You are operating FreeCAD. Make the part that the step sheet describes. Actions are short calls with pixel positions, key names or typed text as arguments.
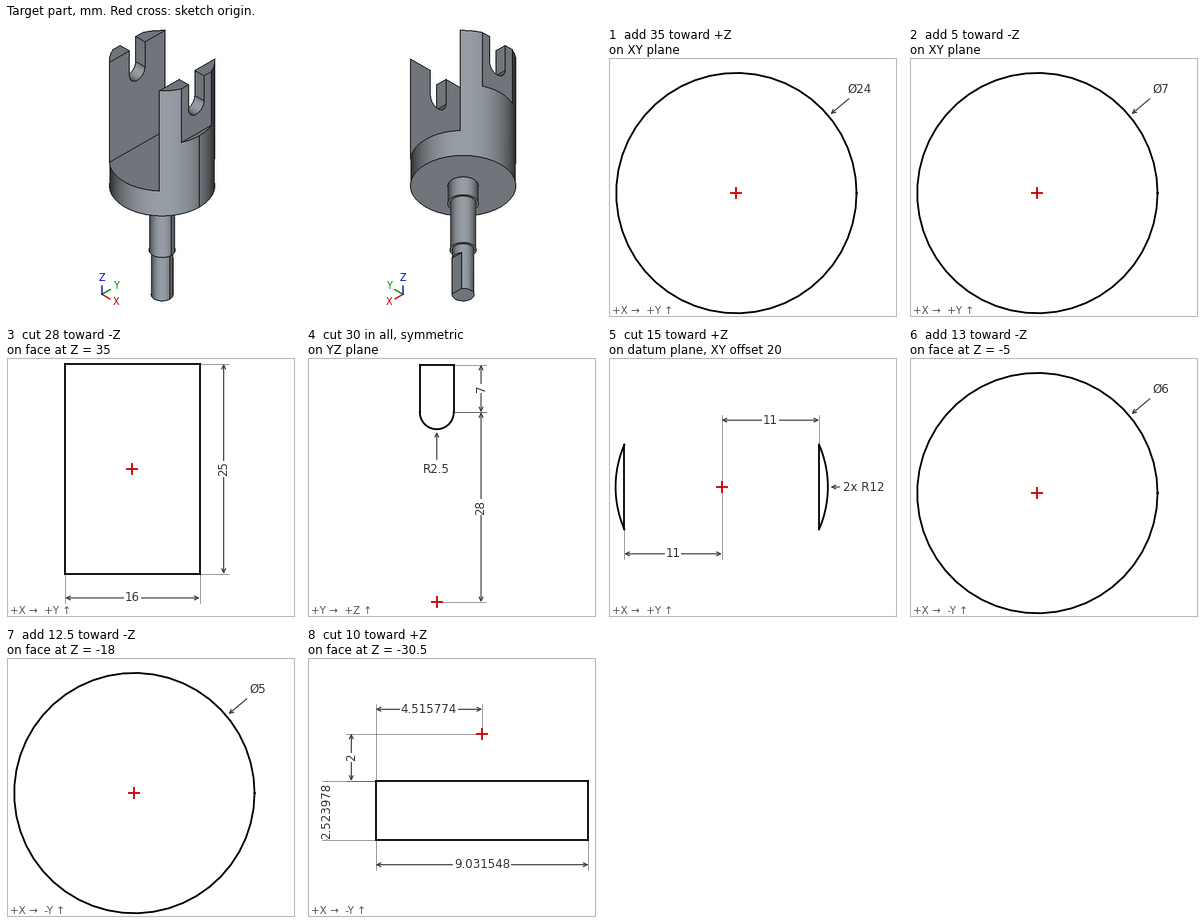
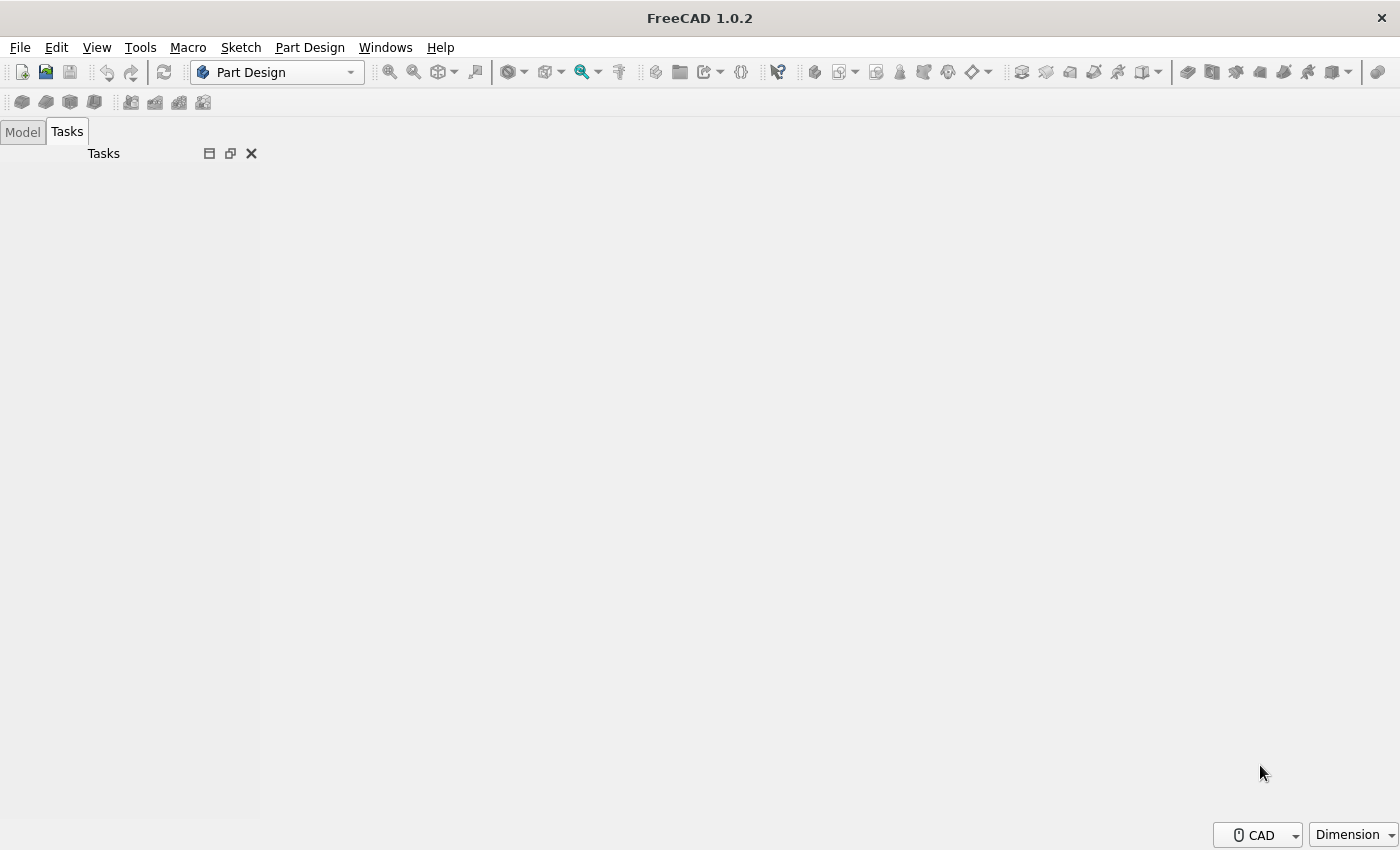
click(22, 72)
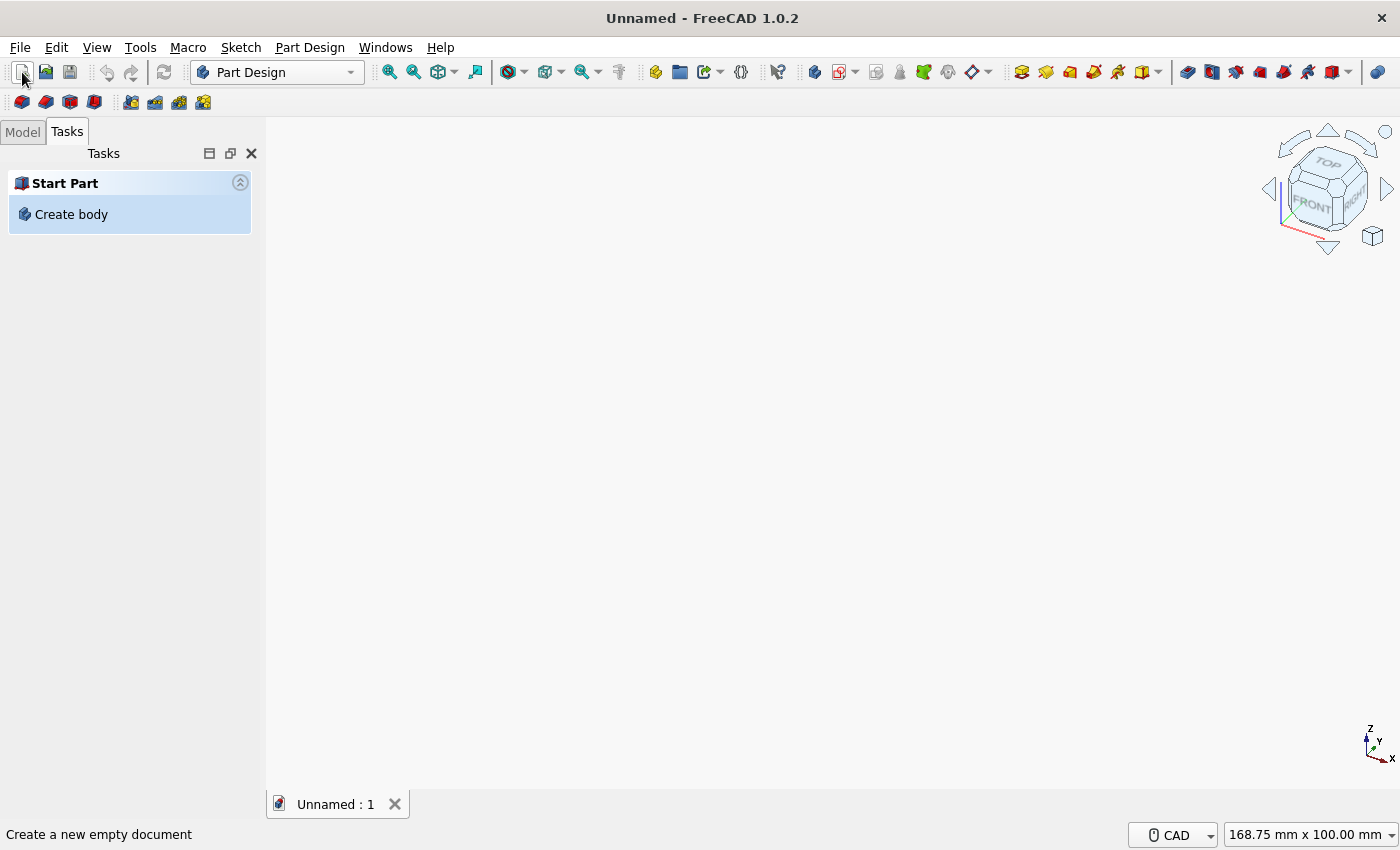
click(840, 72)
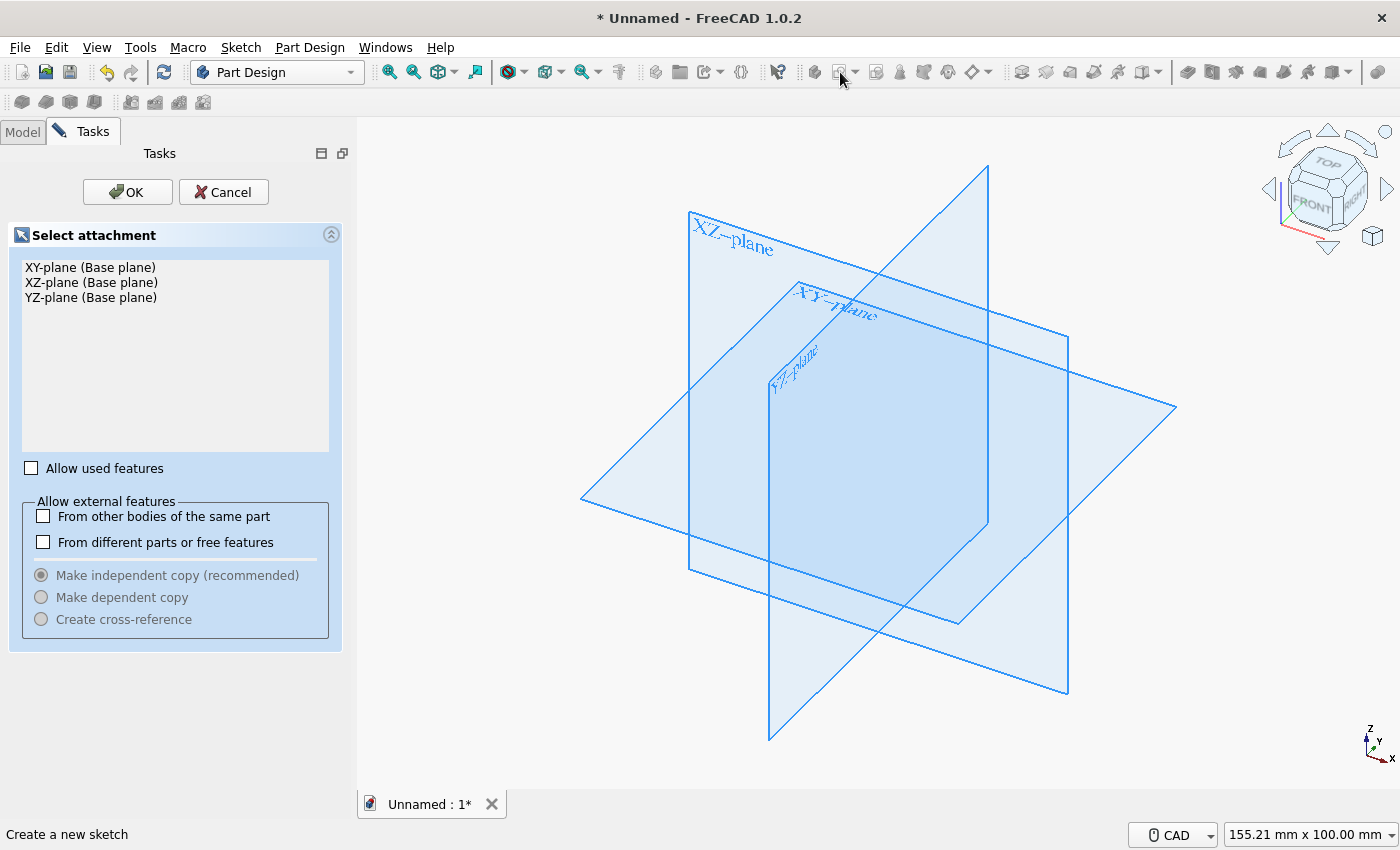
click(82, 268)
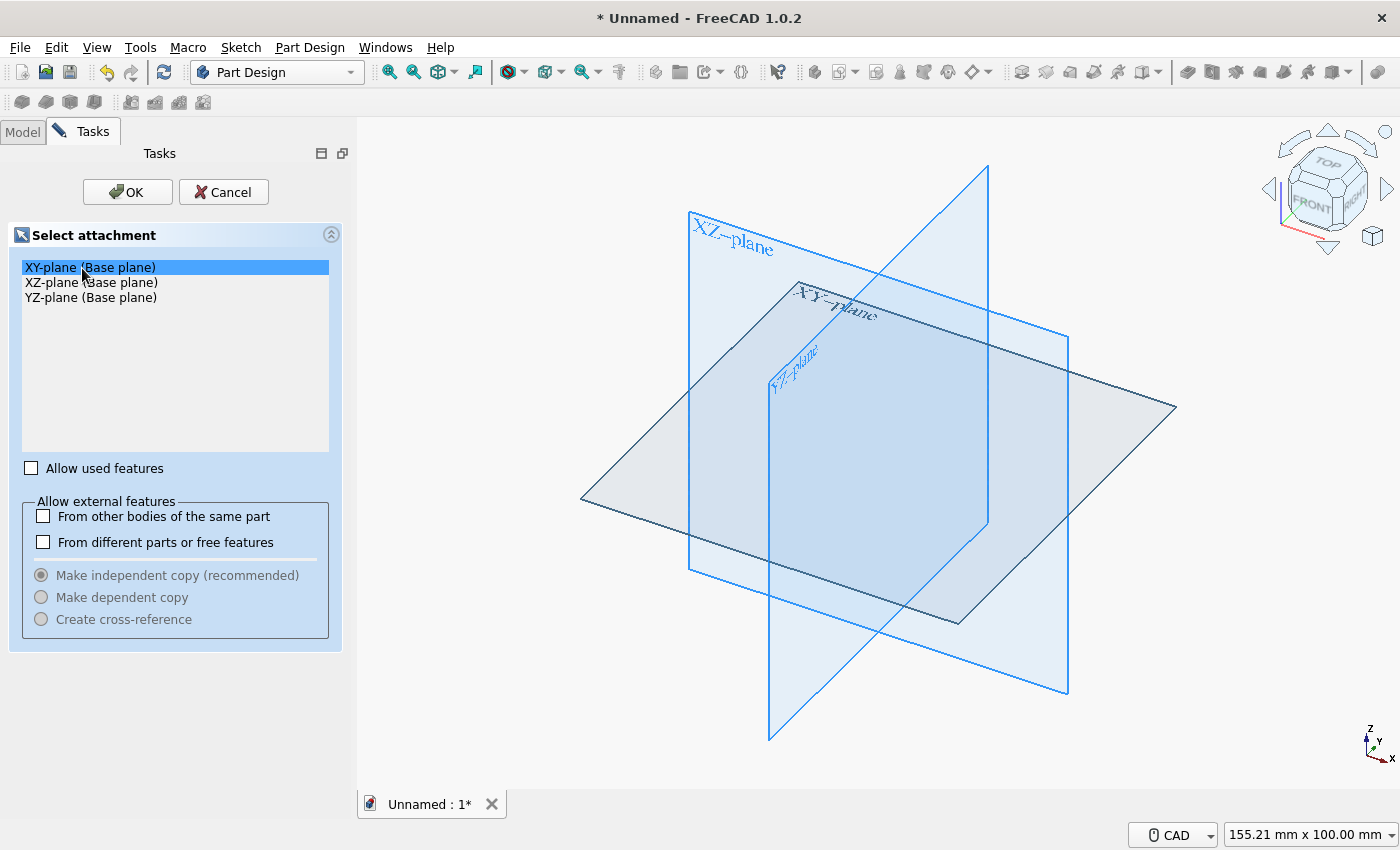
click(128, 192)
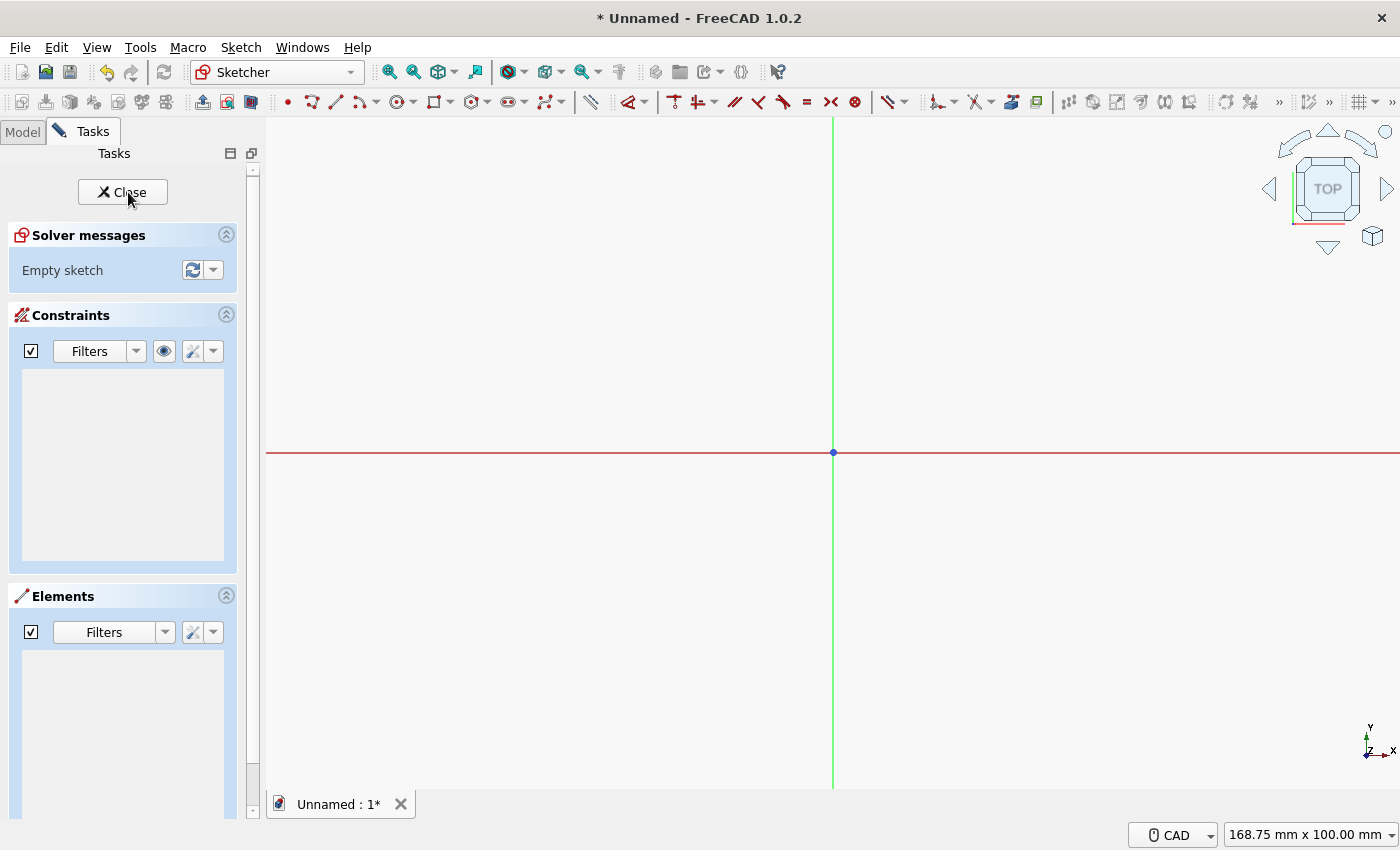
scroll(873, 453, up, 5)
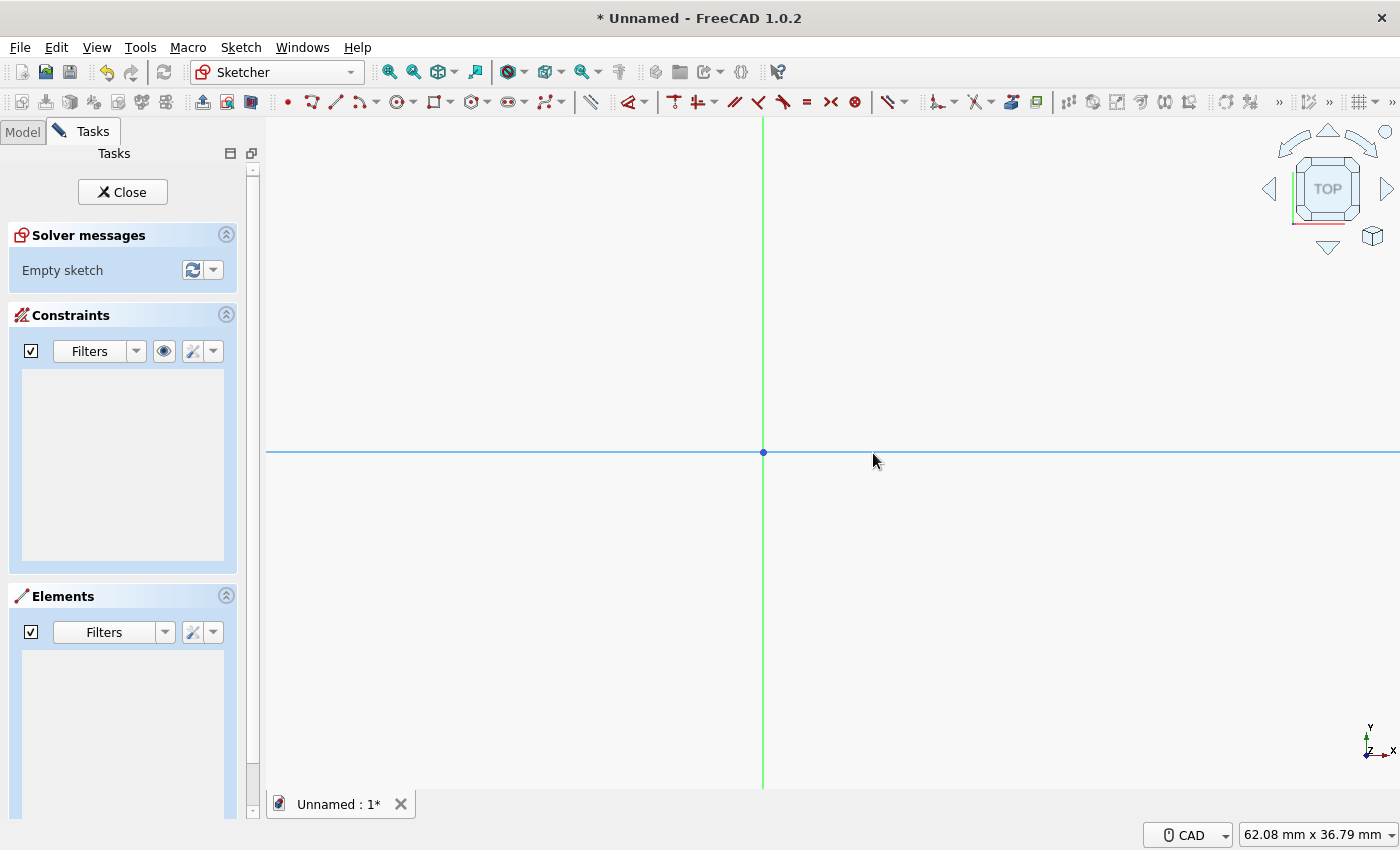
key(g)
key(c)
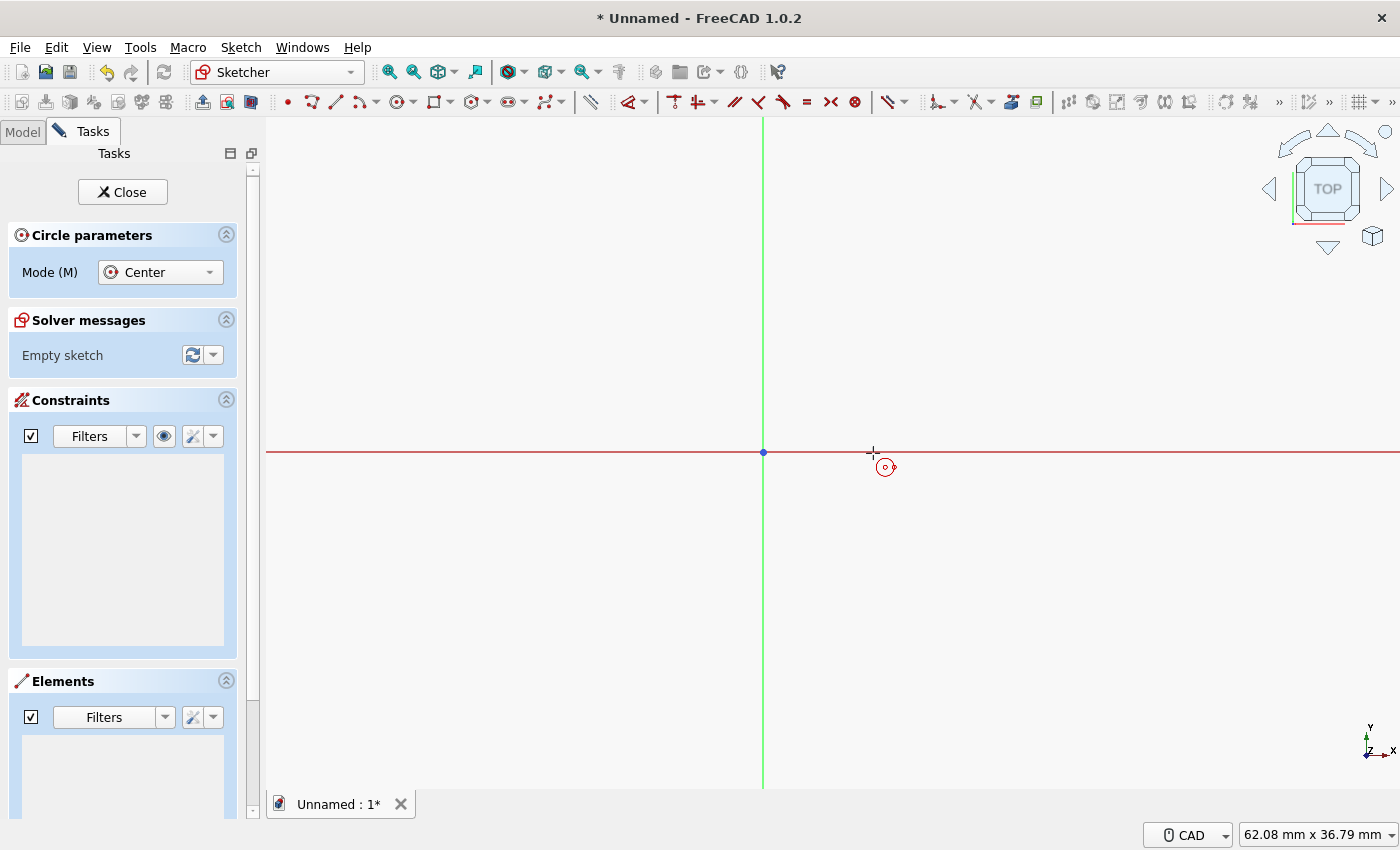
click(763, 452)
click(918, 297)
key(Escape)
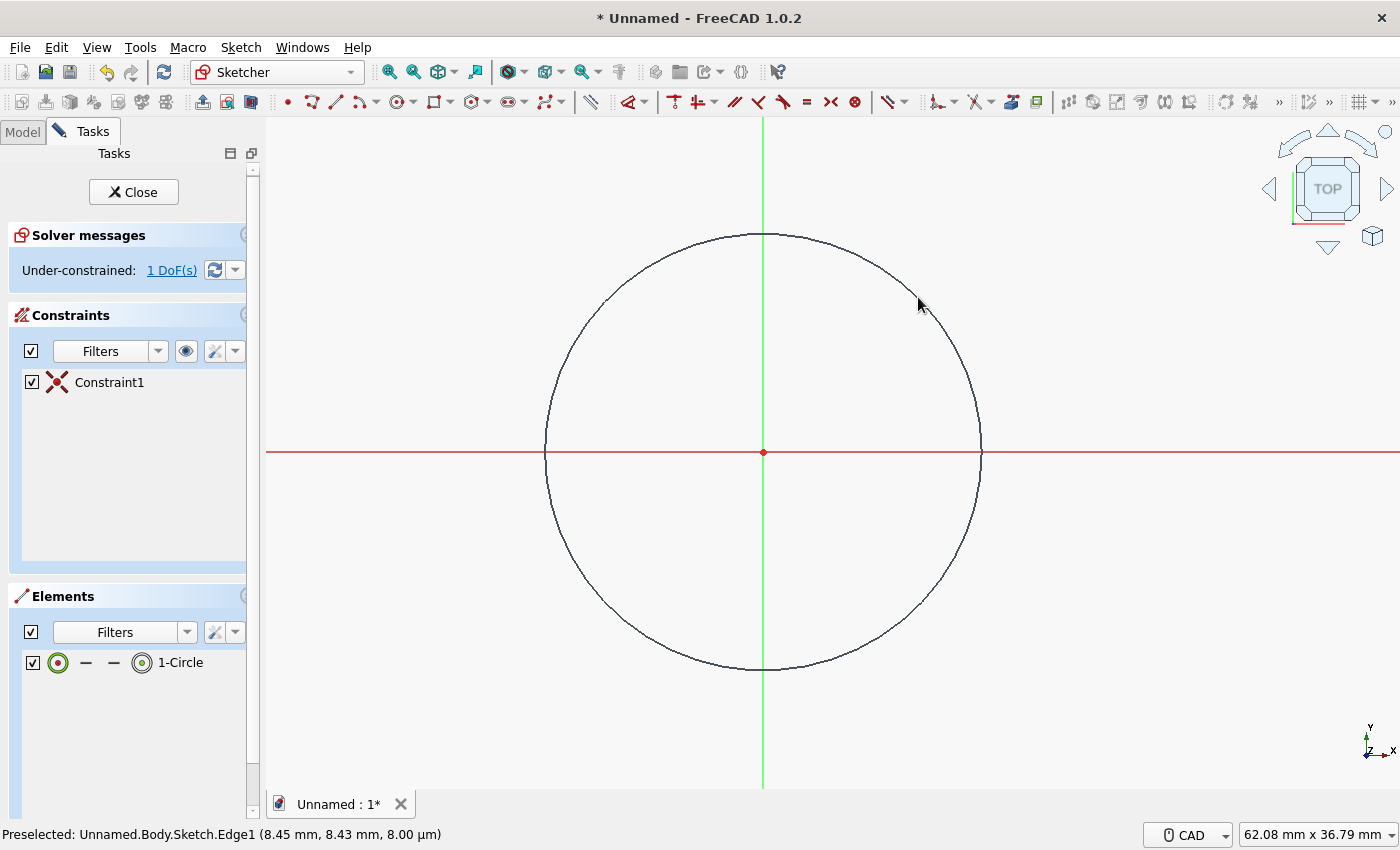
key(d)